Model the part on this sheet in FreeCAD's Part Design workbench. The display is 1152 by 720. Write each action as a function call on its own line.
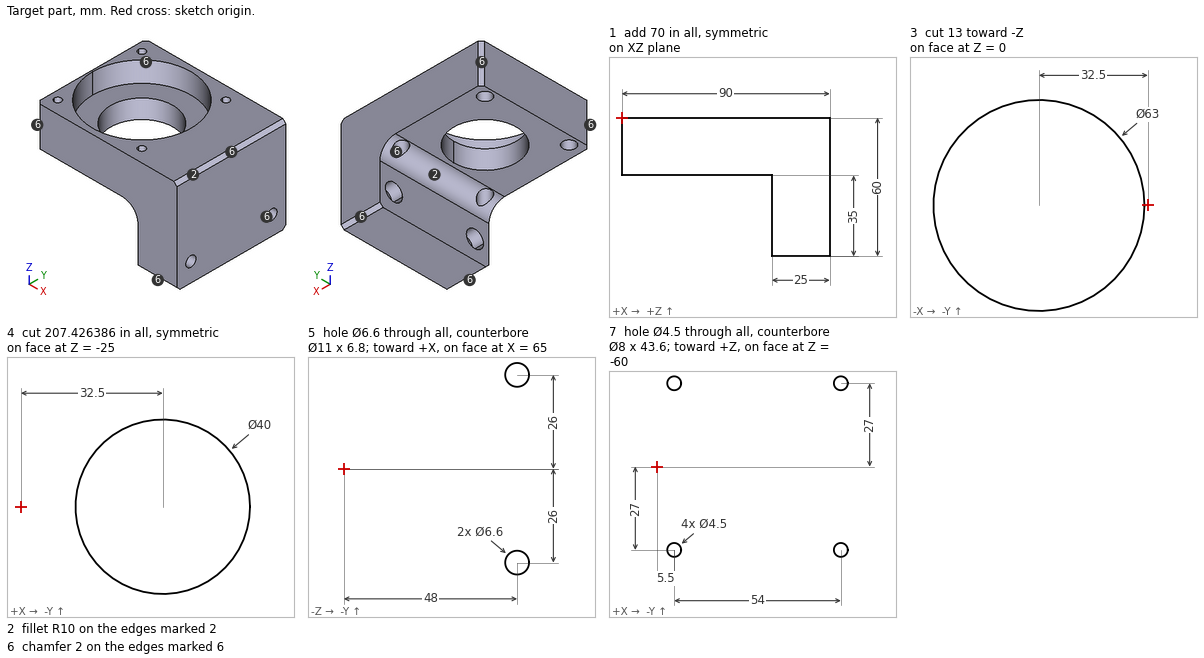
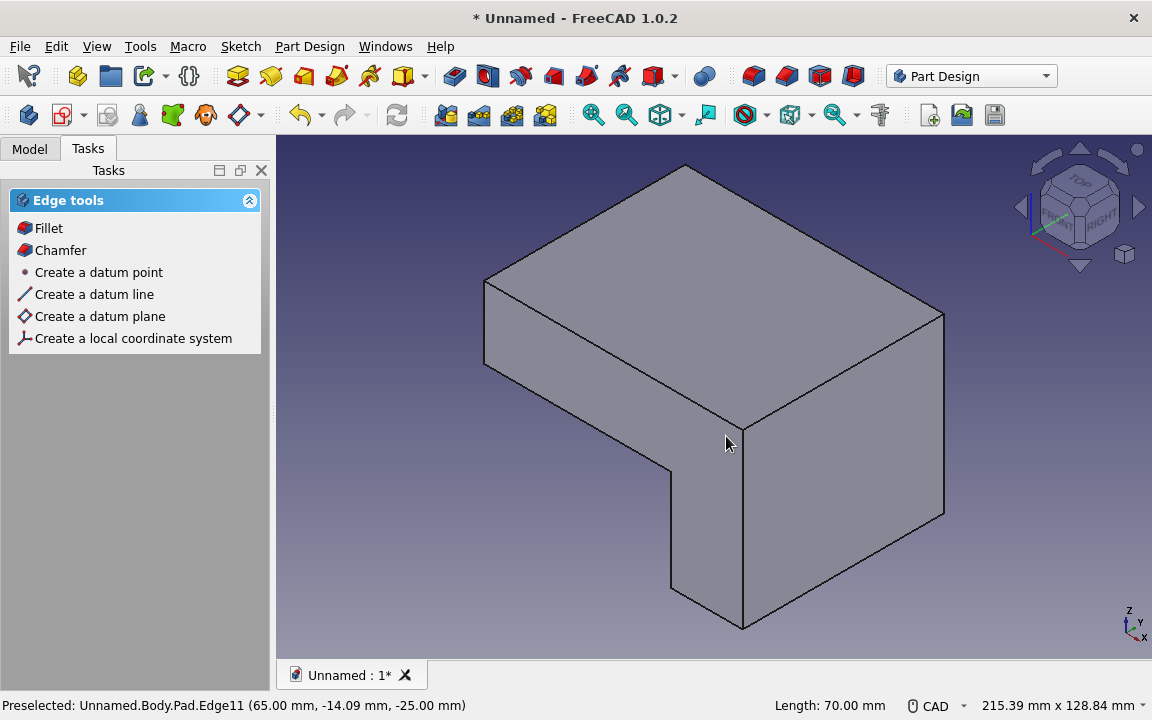
click(754, 76)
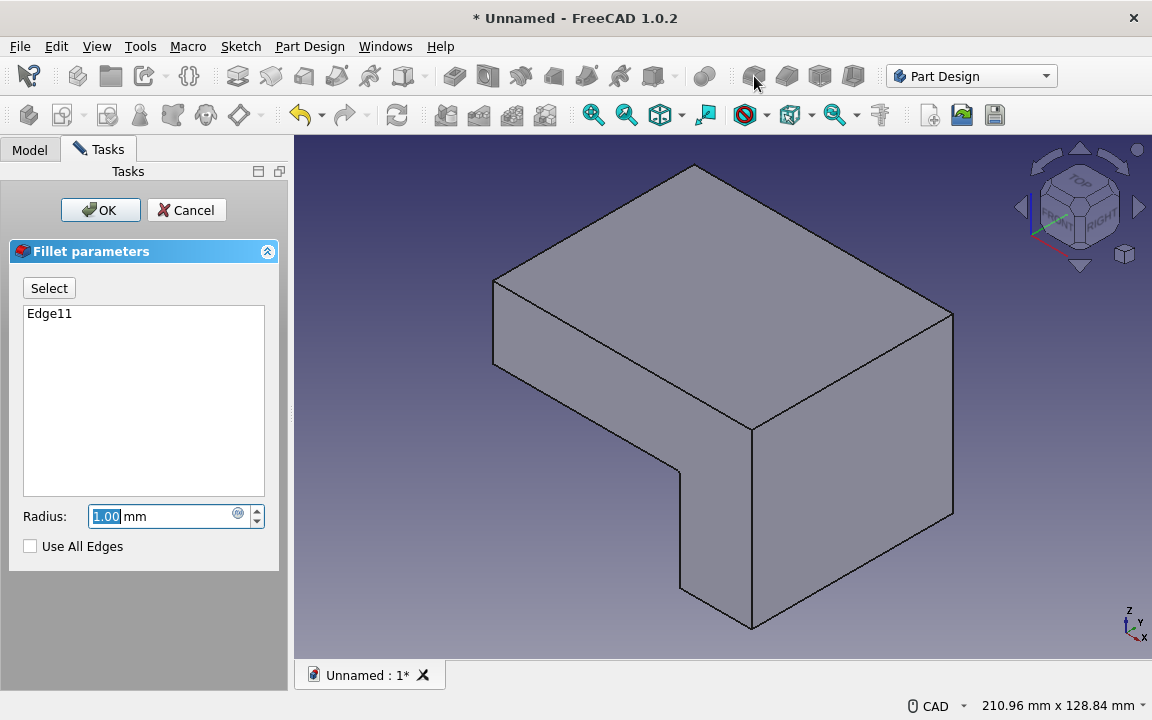
text(10)
key(Tab)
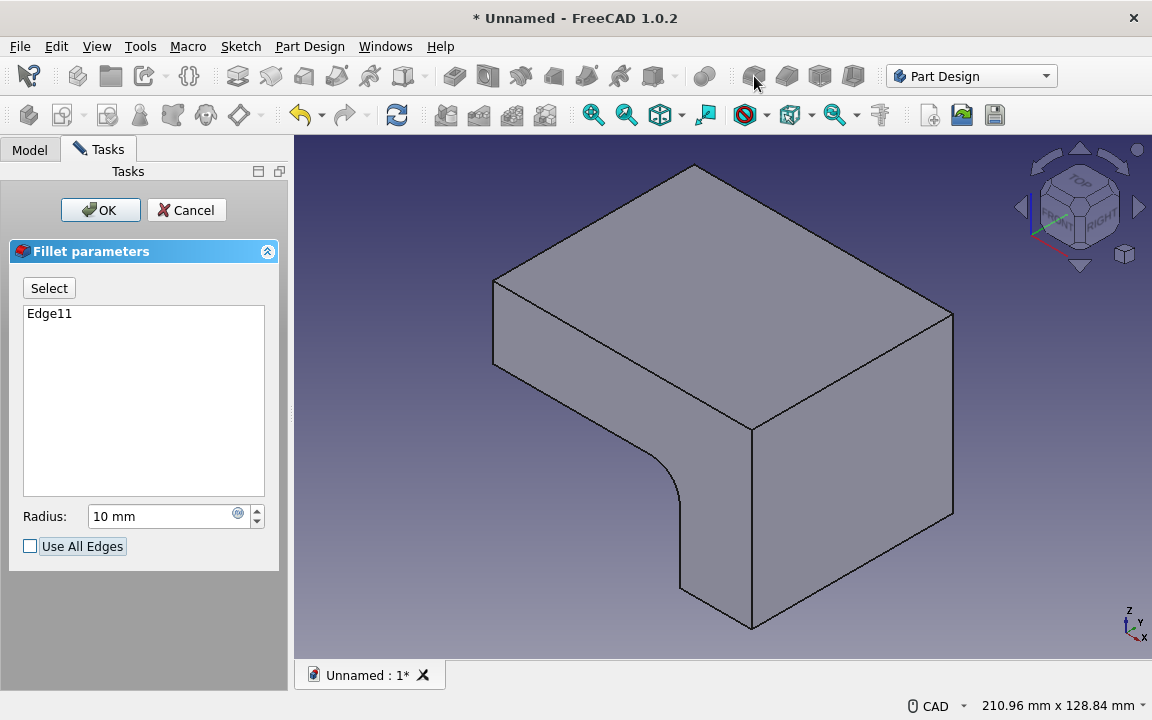
click(101, 210)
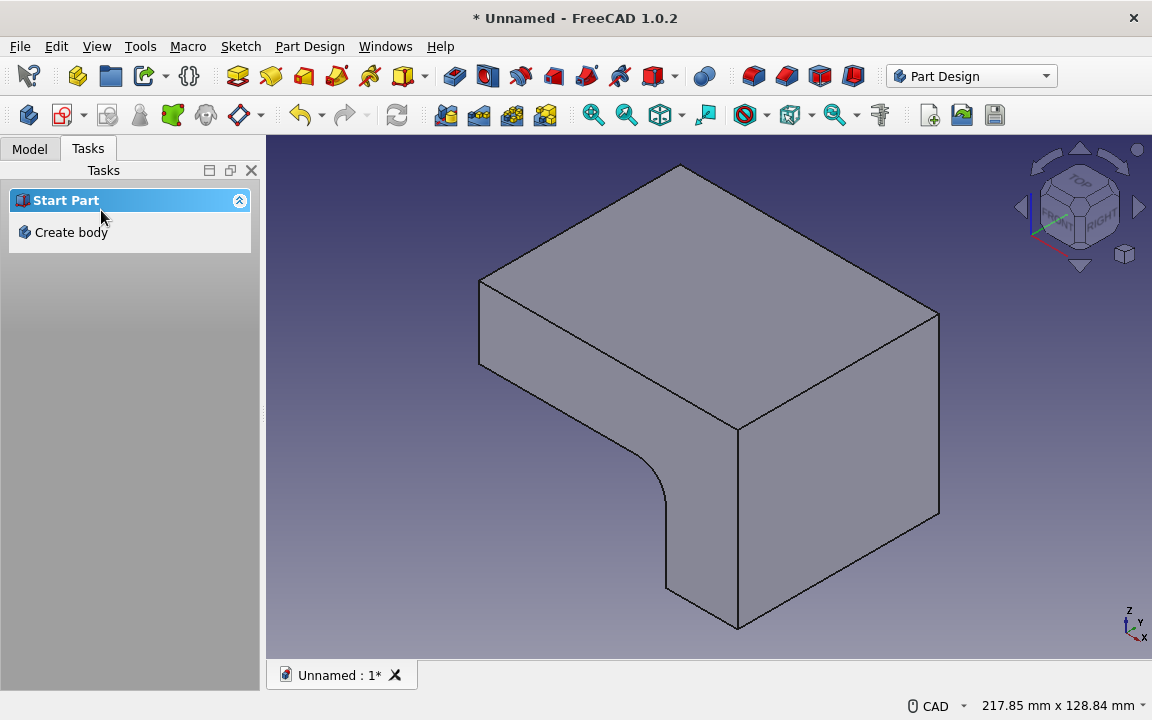
click(709, 296)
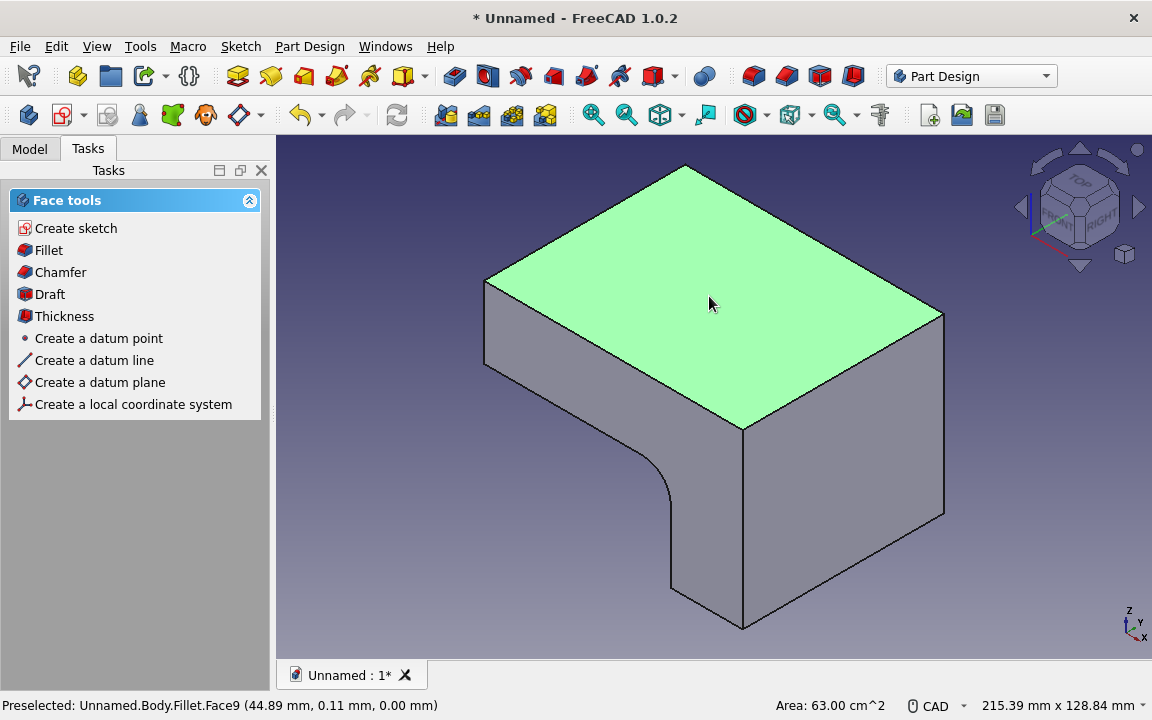
click(62, 116)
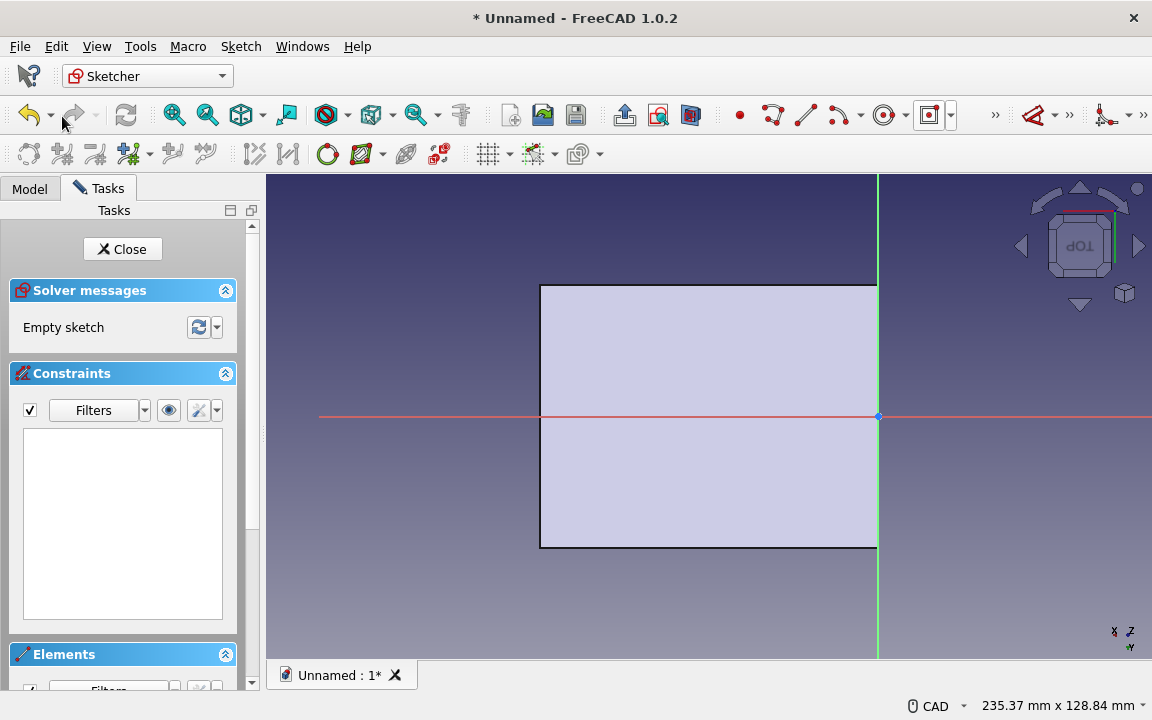
click(884, 116)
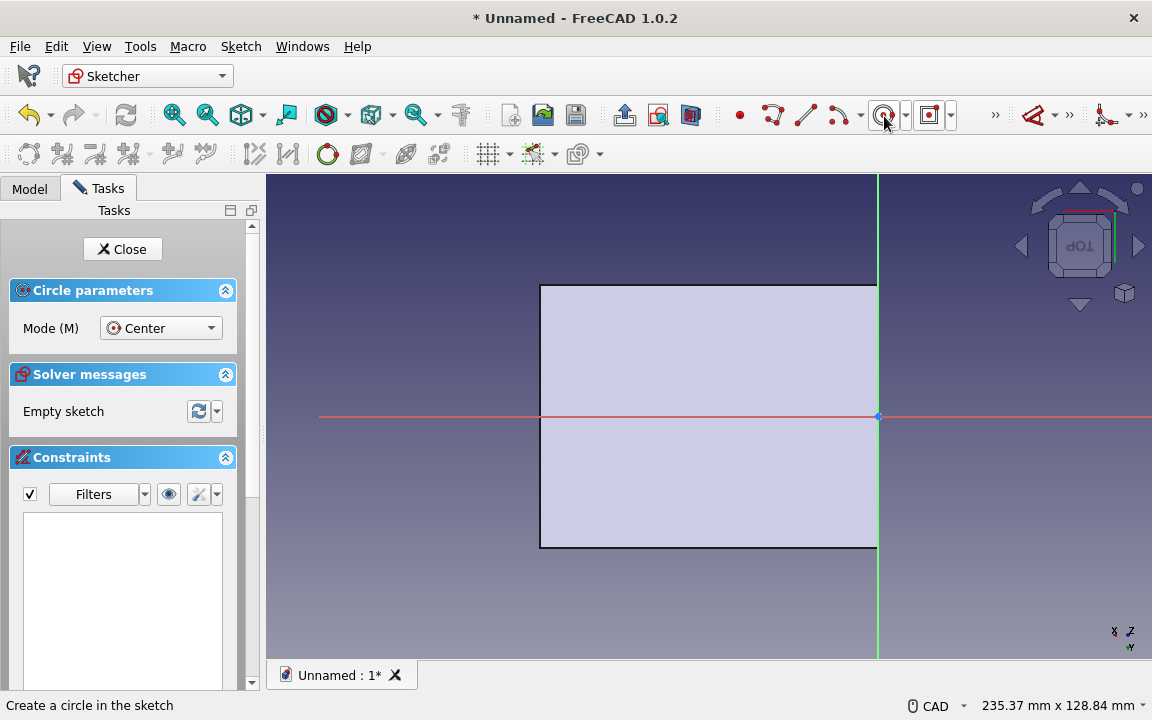
click(756, 416)
move(840, 333)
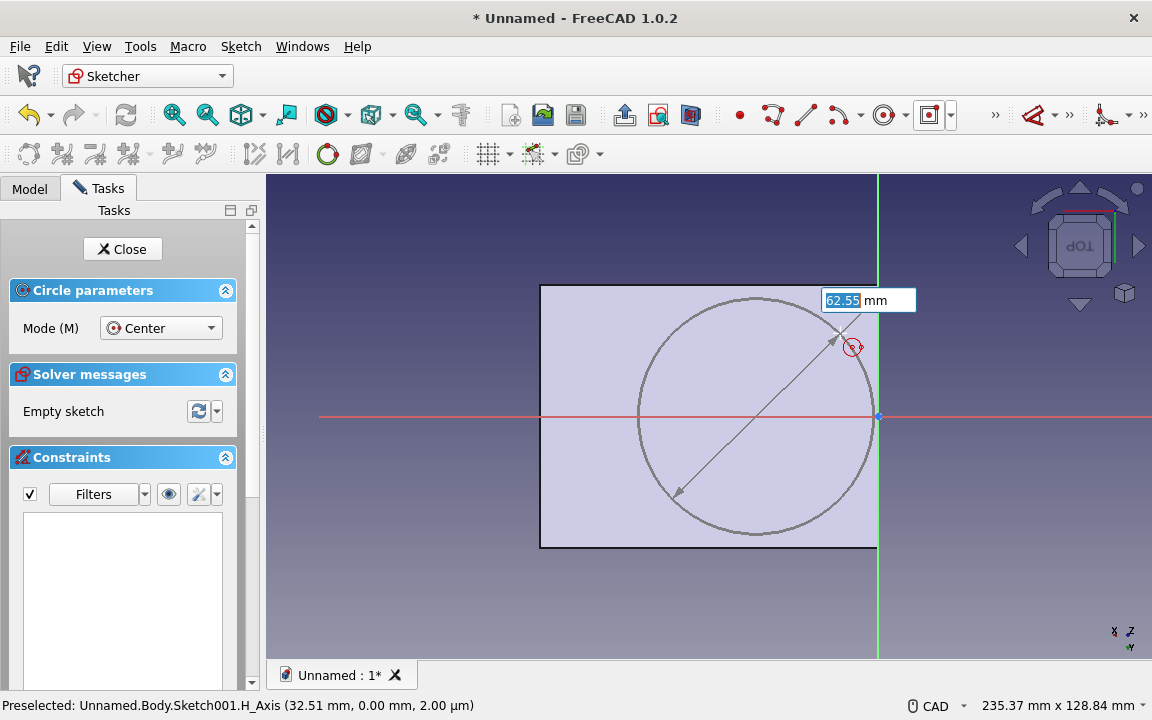
text(63)
key(Return)
key(Escape)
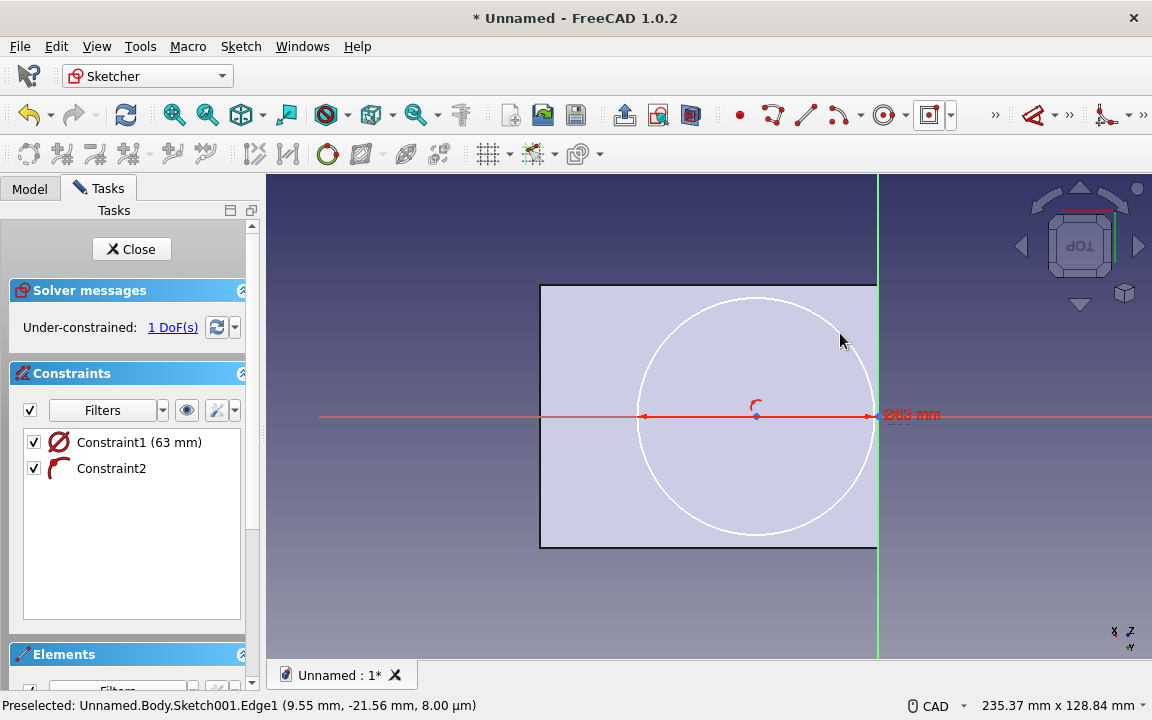
click(1032, 116)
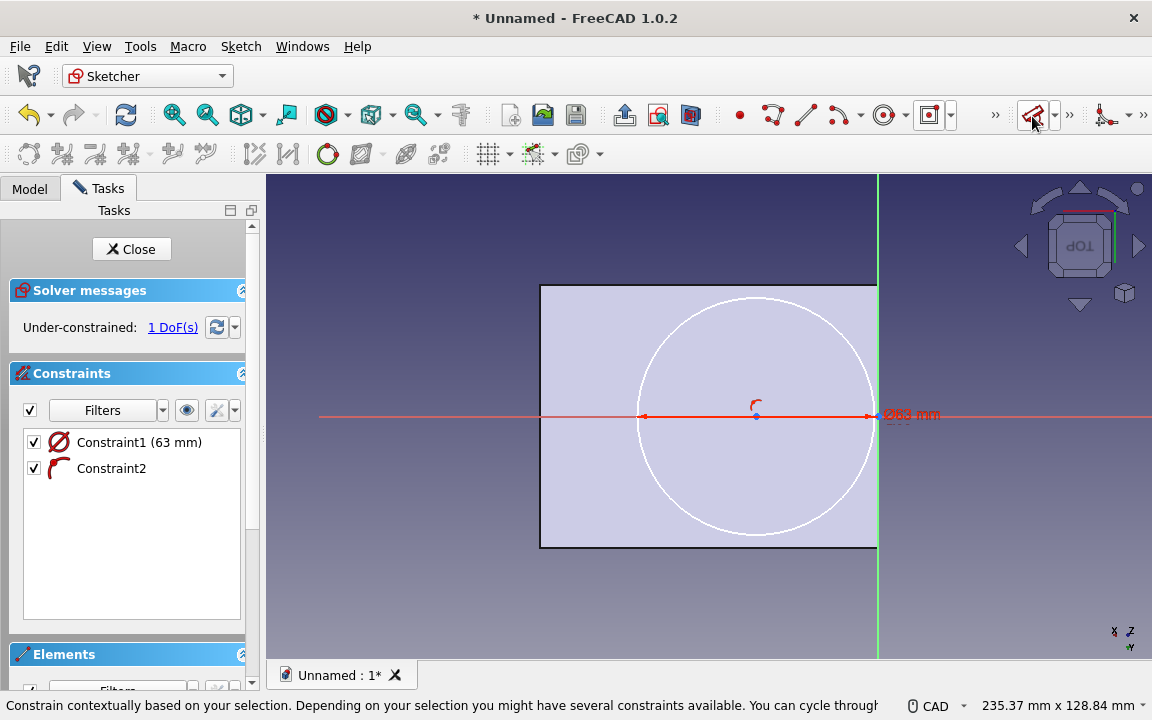
click(756, 416)
click(817, 450)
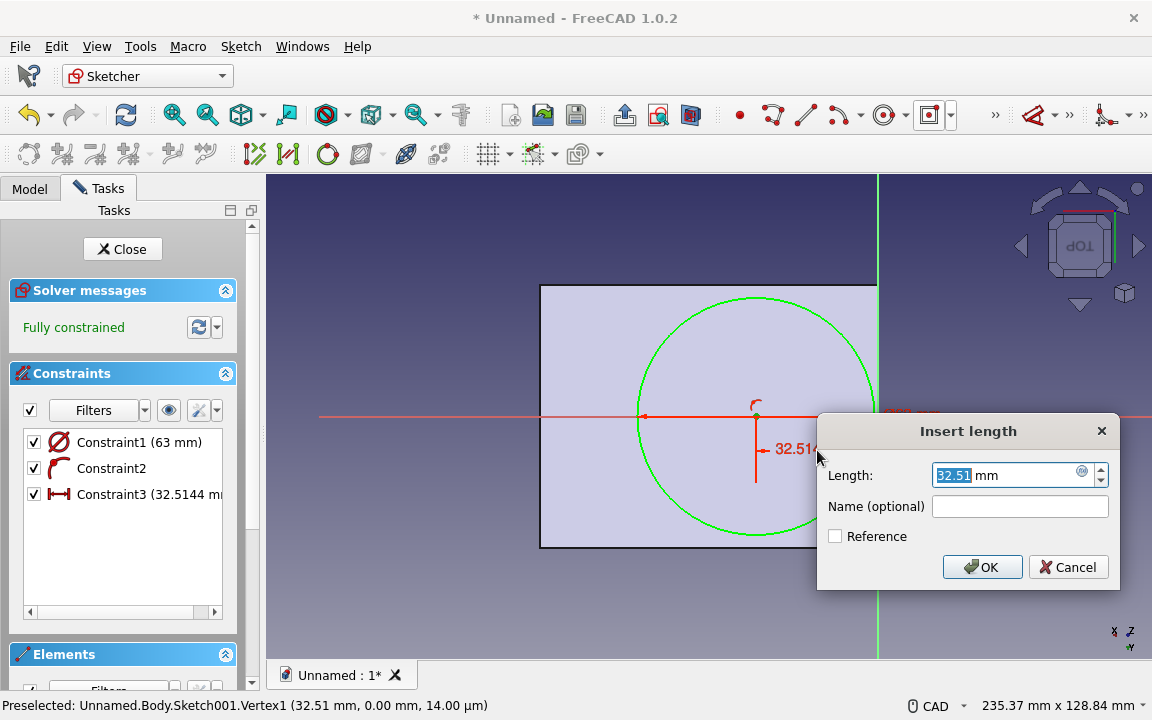
text(32.5)
key(Return)
key(Escape)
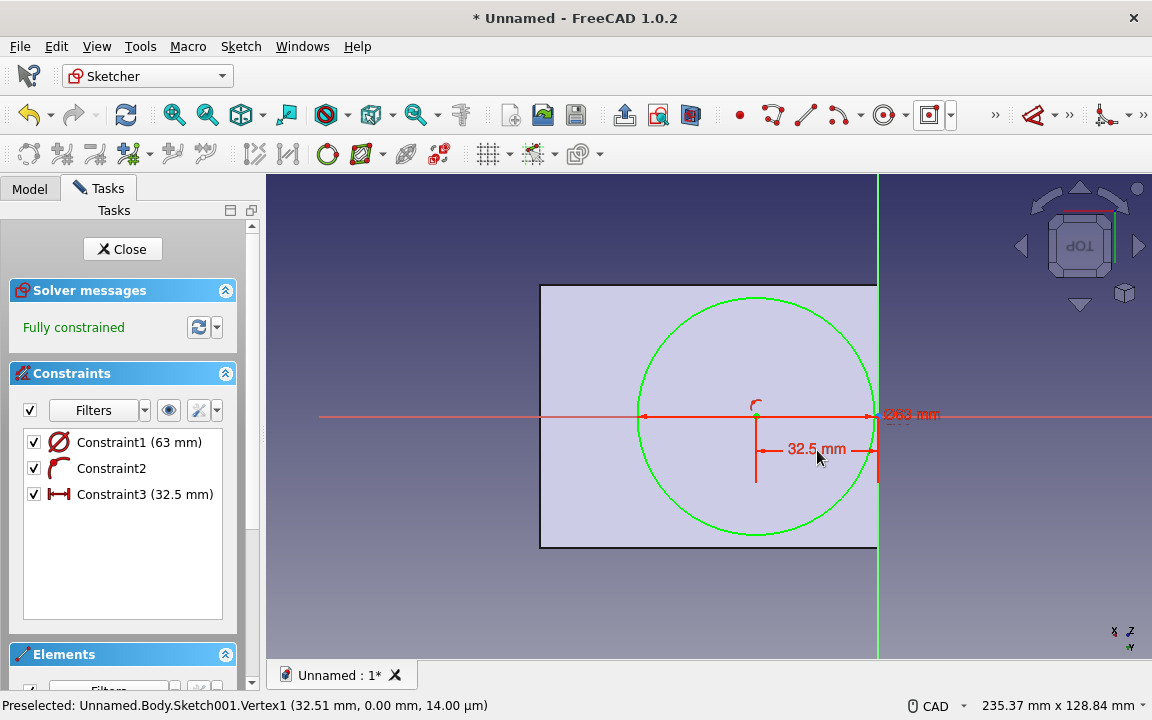
click(123, 249)